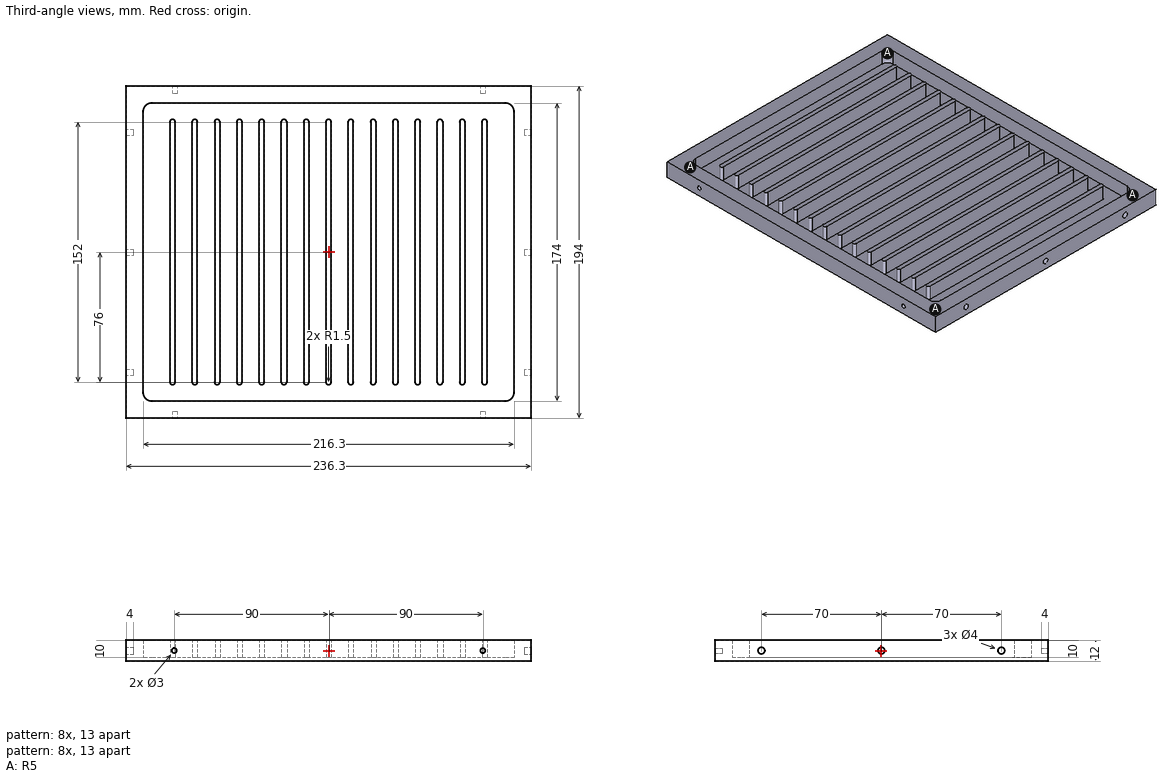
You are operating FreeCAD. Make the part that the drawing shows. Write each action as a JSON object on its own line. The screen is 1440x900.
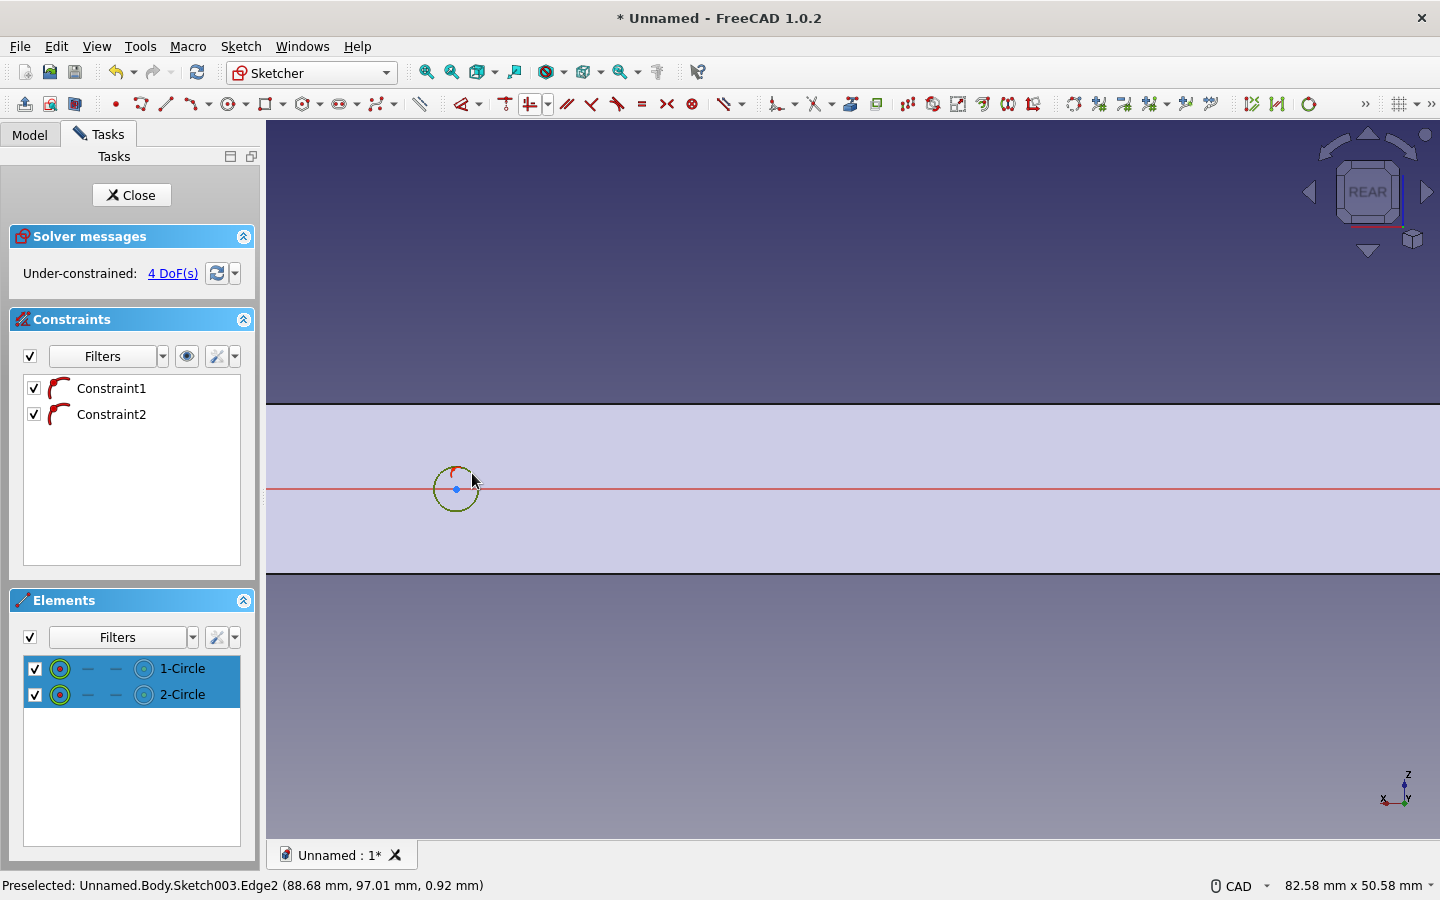
{"action": "left_click", "coordinate": [642, 104]}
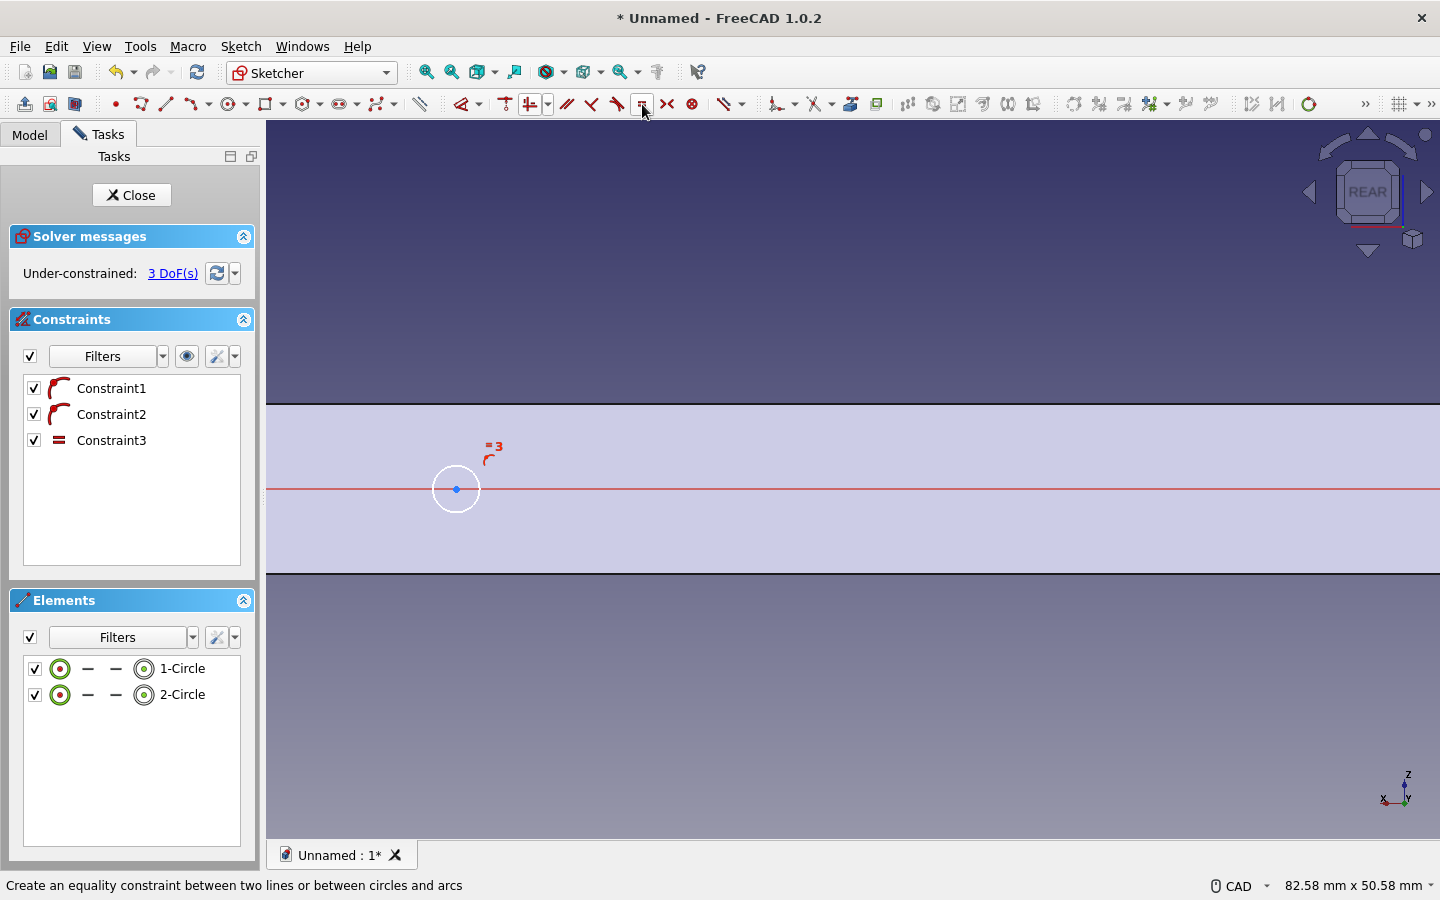
{"action": "left_click", "coordinate": [460, 104]}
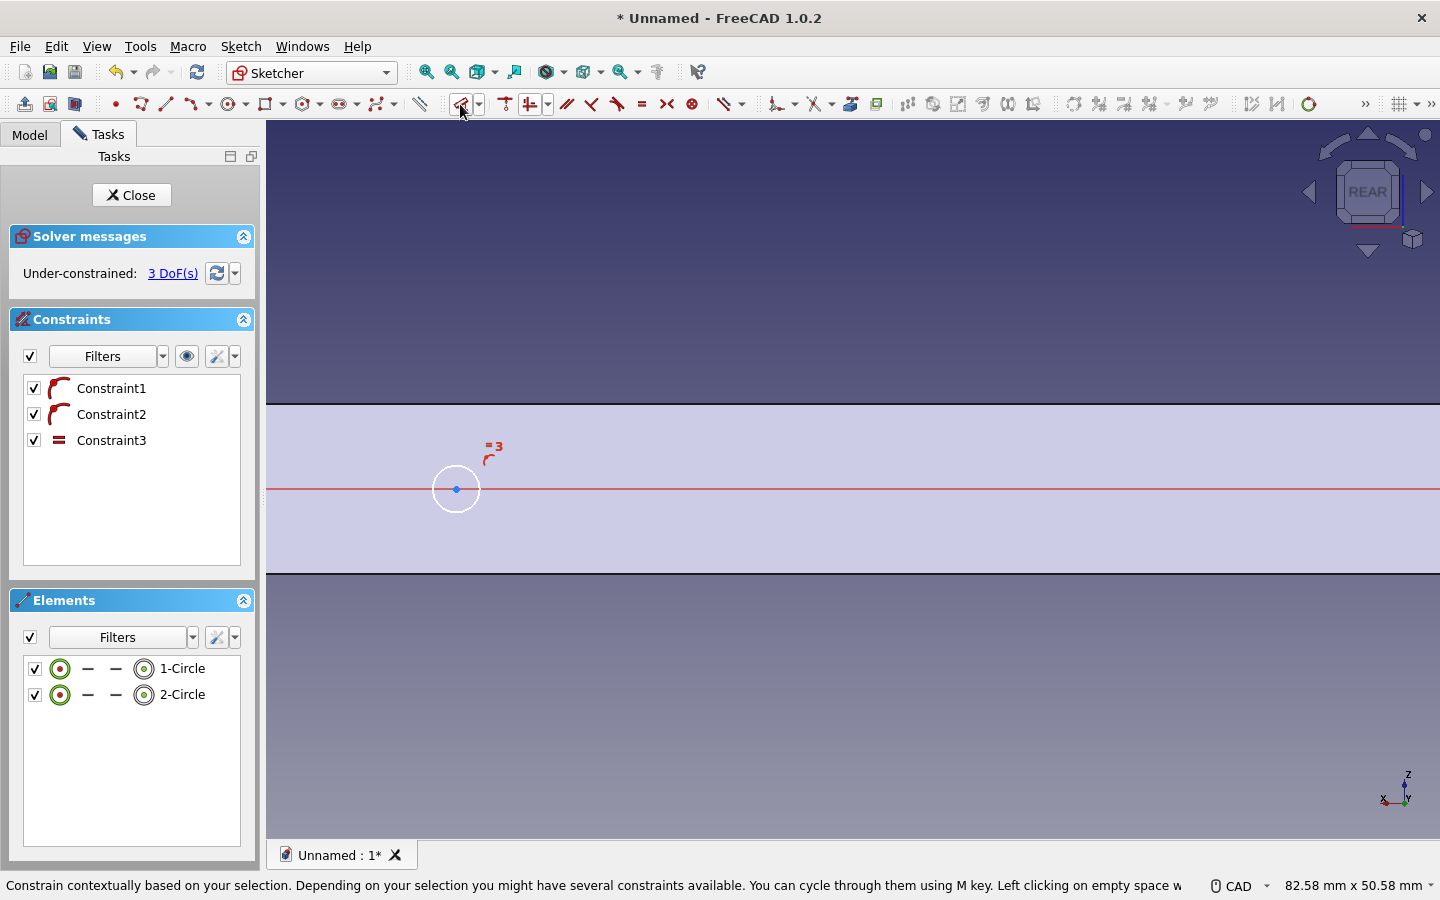
{"action": "scroll", "coordinate": [473, 476], "scroll_direction": "down", "scroll_amount": 7}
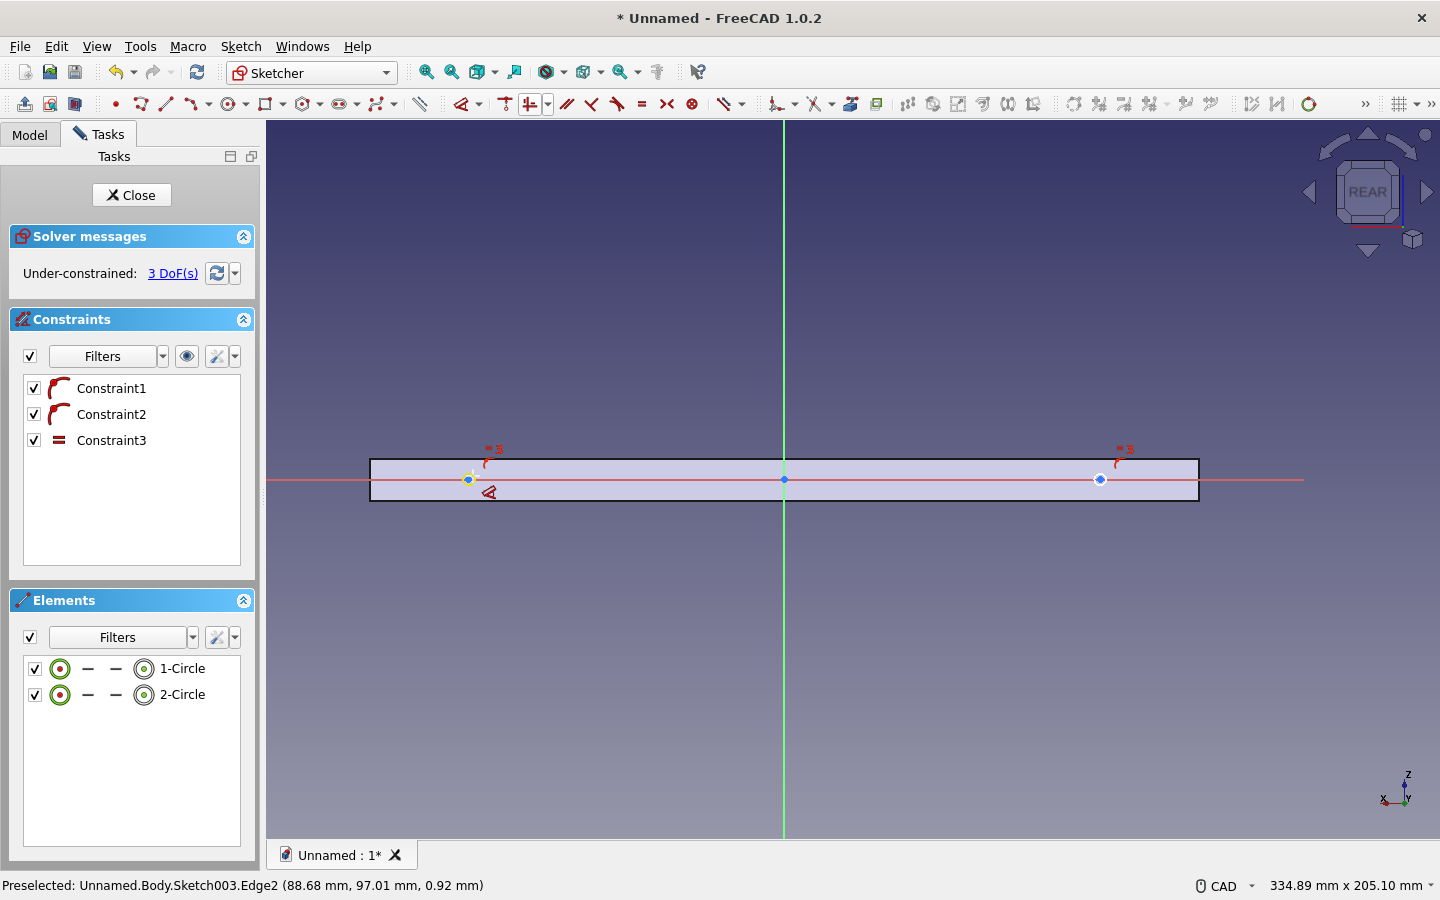
{"action": "scroll", "coordinate": [1104, 476], "scroll_direction": "up", "scroll_amount": 7}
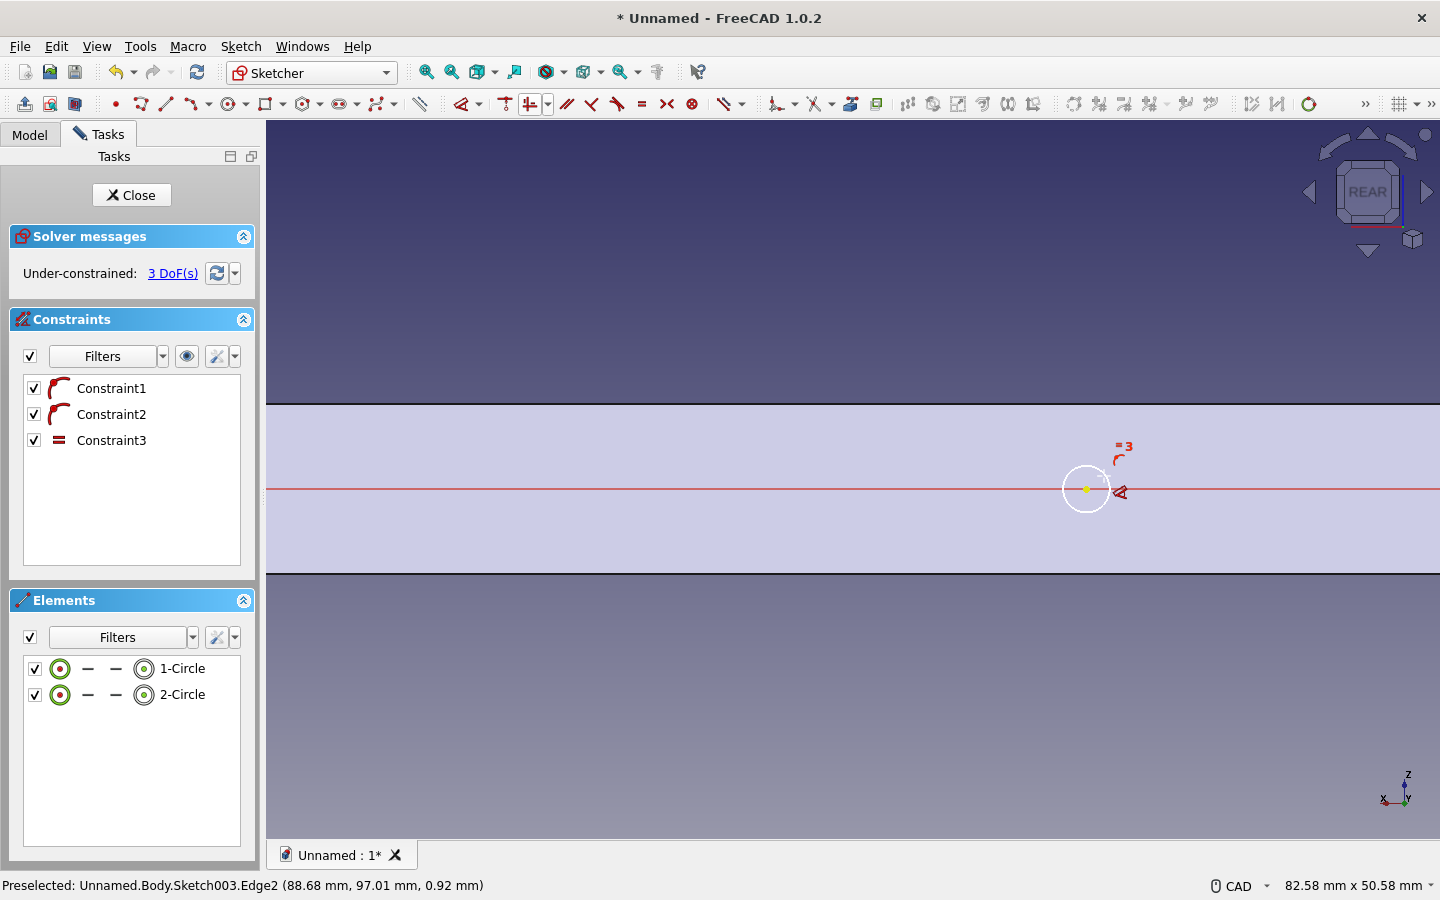
{"action": "left_click", "coordinate": [1103, 473]}
{"action": "left_click", "coordinate": [1126, 451]}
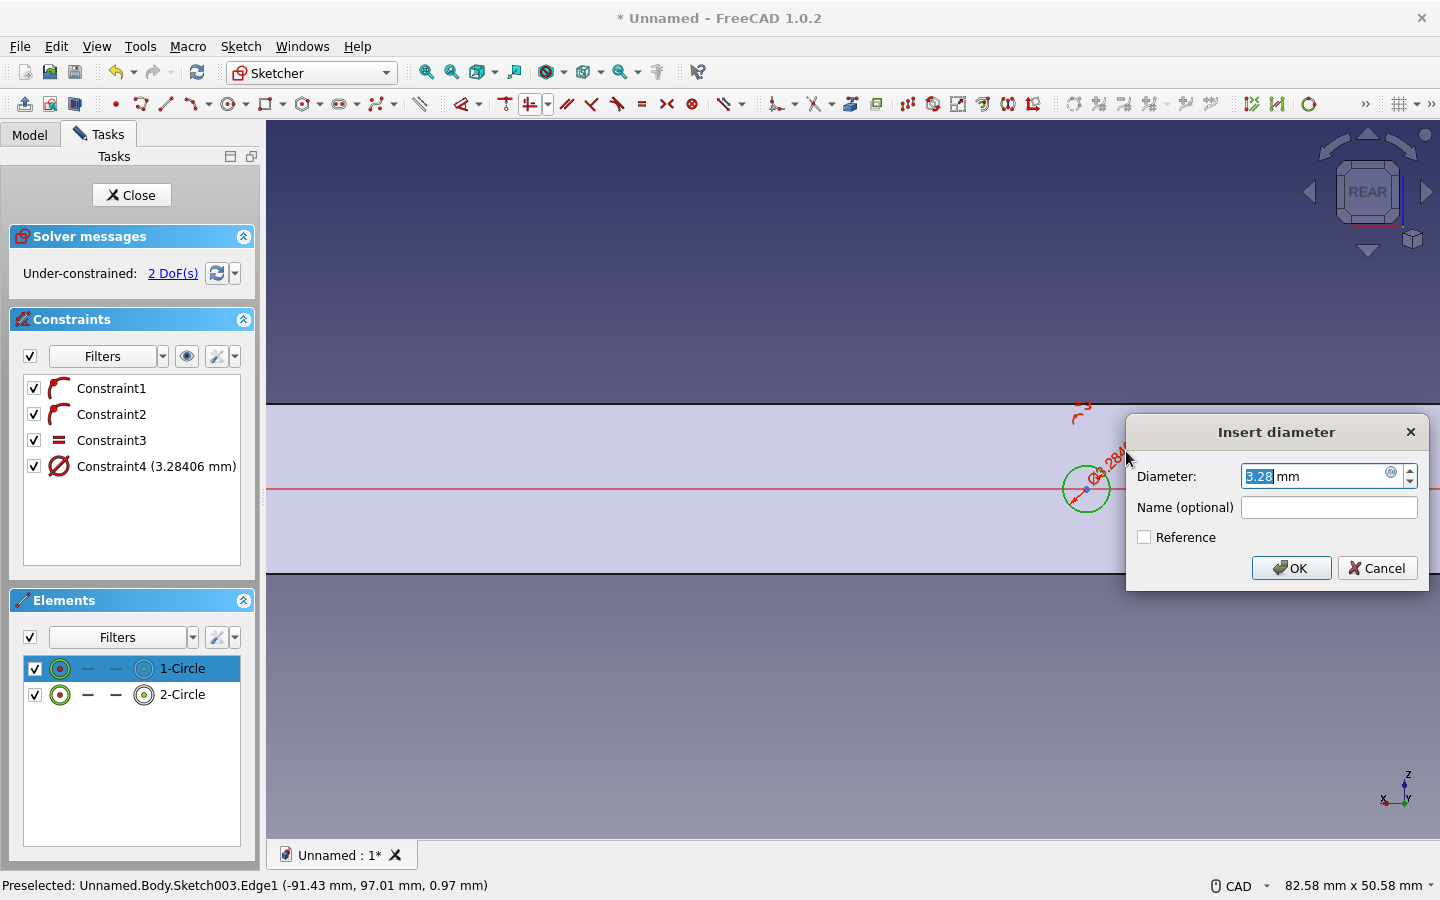
{"action": "type", "text": "3"}
{"action": "key", "text": "Return"}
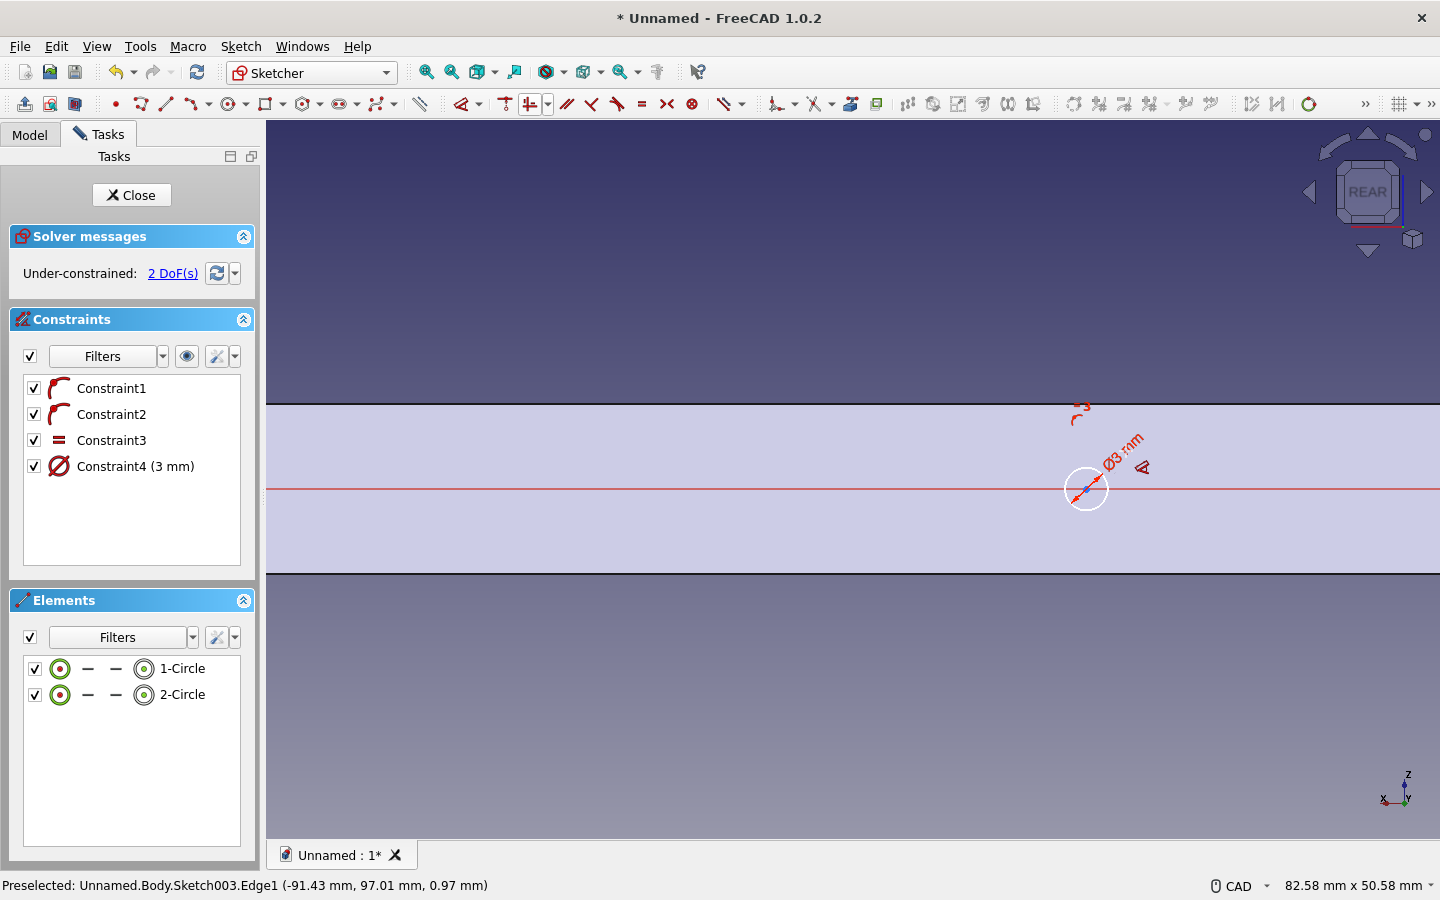
{"action": "scroll", "coordinate": [1105, 476], "scroll_direction": "down", "scroll_amount": 7}